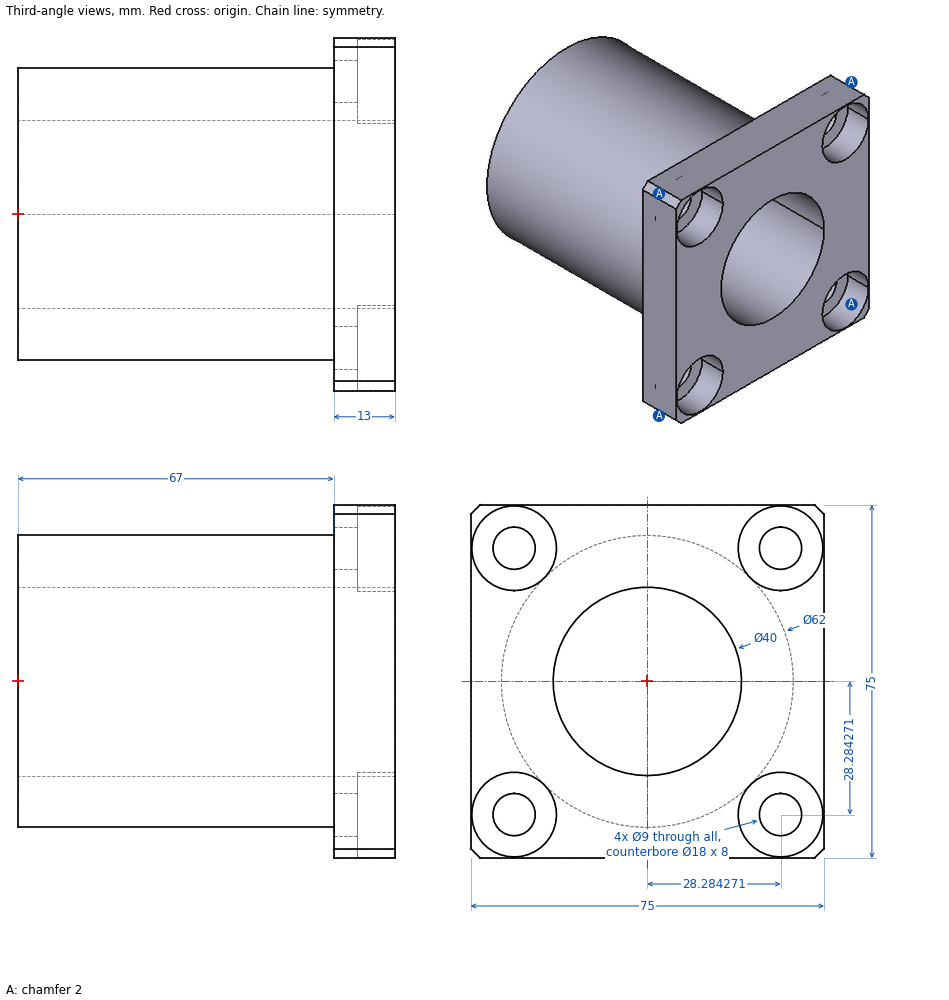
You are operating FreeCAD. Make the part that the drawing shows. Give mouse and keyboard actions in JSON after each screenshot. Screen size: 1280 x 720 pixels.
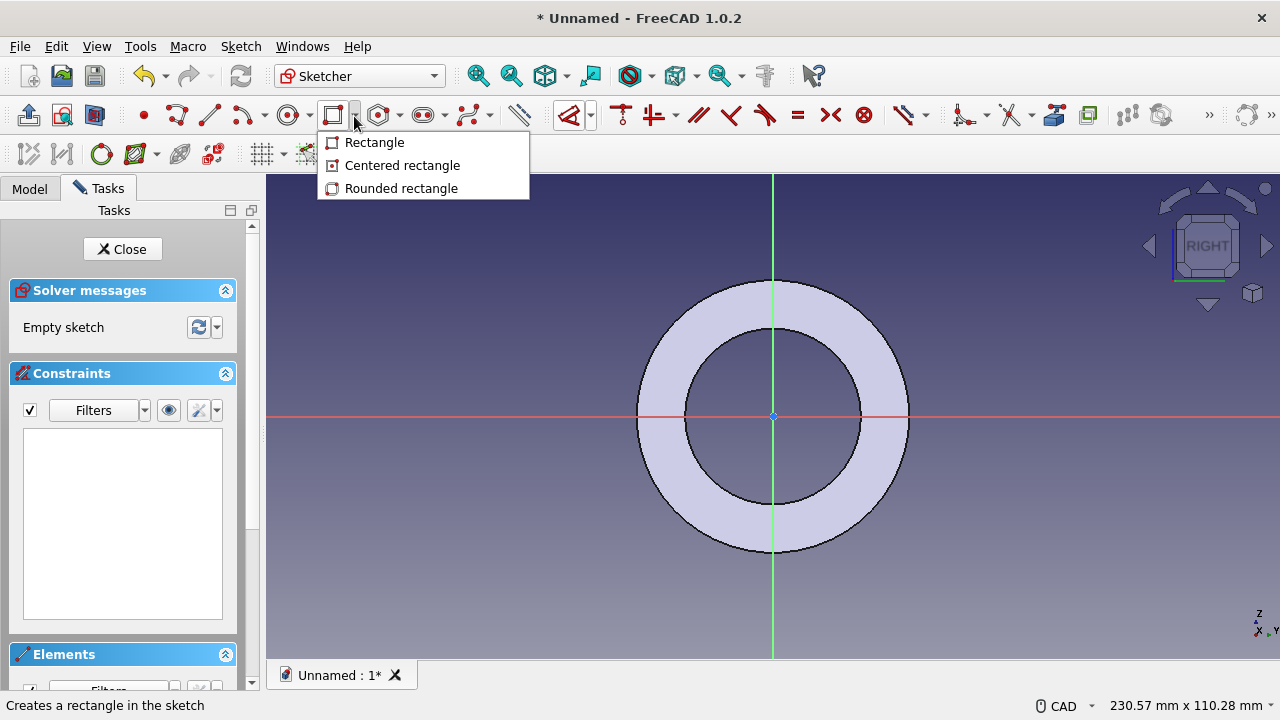
{"action": "left_click", "coordinate": [424, 166]}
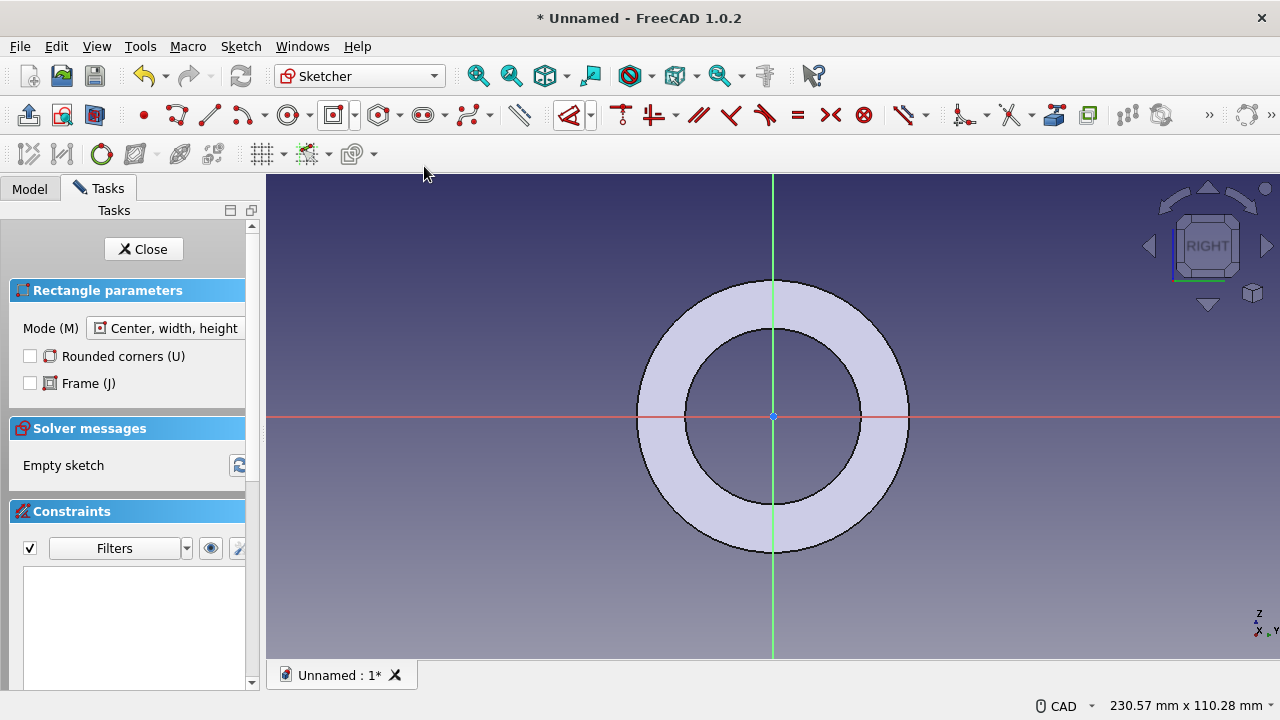
{"action": "left_click", "coordinate": [773, 416]}
{"action": "left_click", "coordinate": [938, 252]}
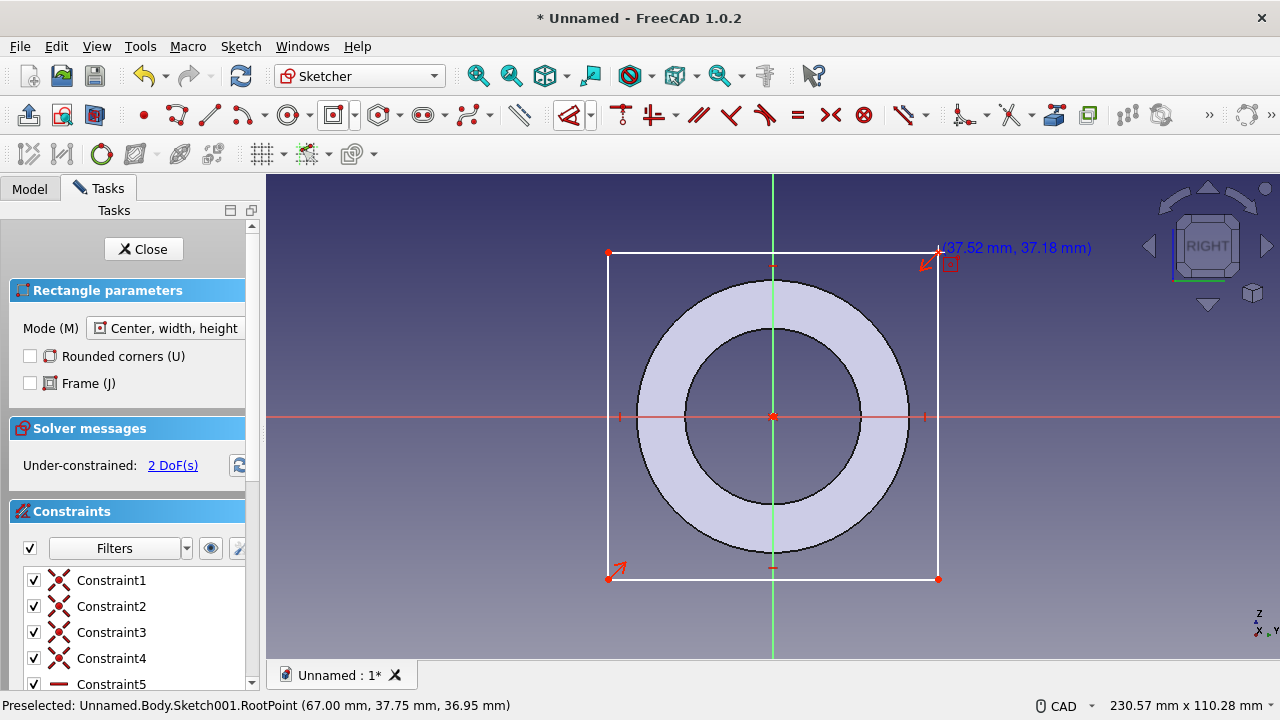
{"action": "left_click", "coordinate": [288, 116]}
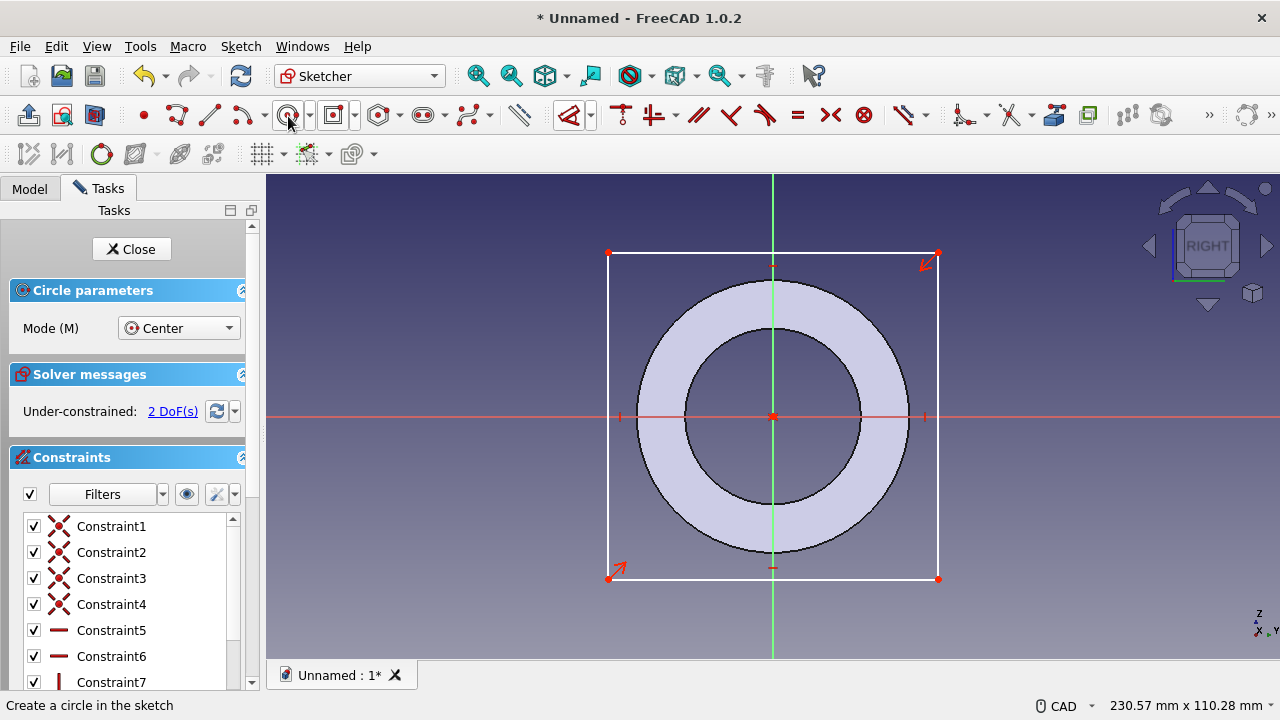
{"action": "left_click", "coordinate": [773, 416]}
{"action": "left_click", "coordinate": [835, 354]}
{"action": "key", "text": "Escape"}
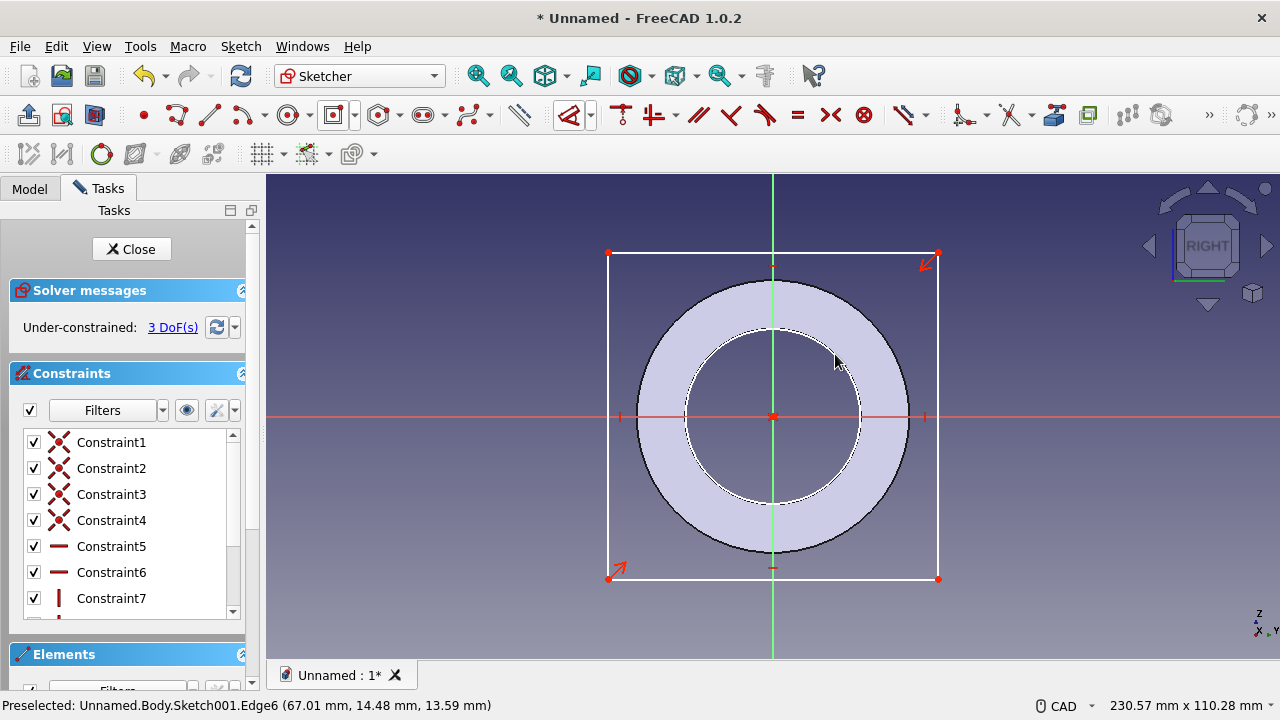
{"action": "left_click", "coordinate": [835, 355]}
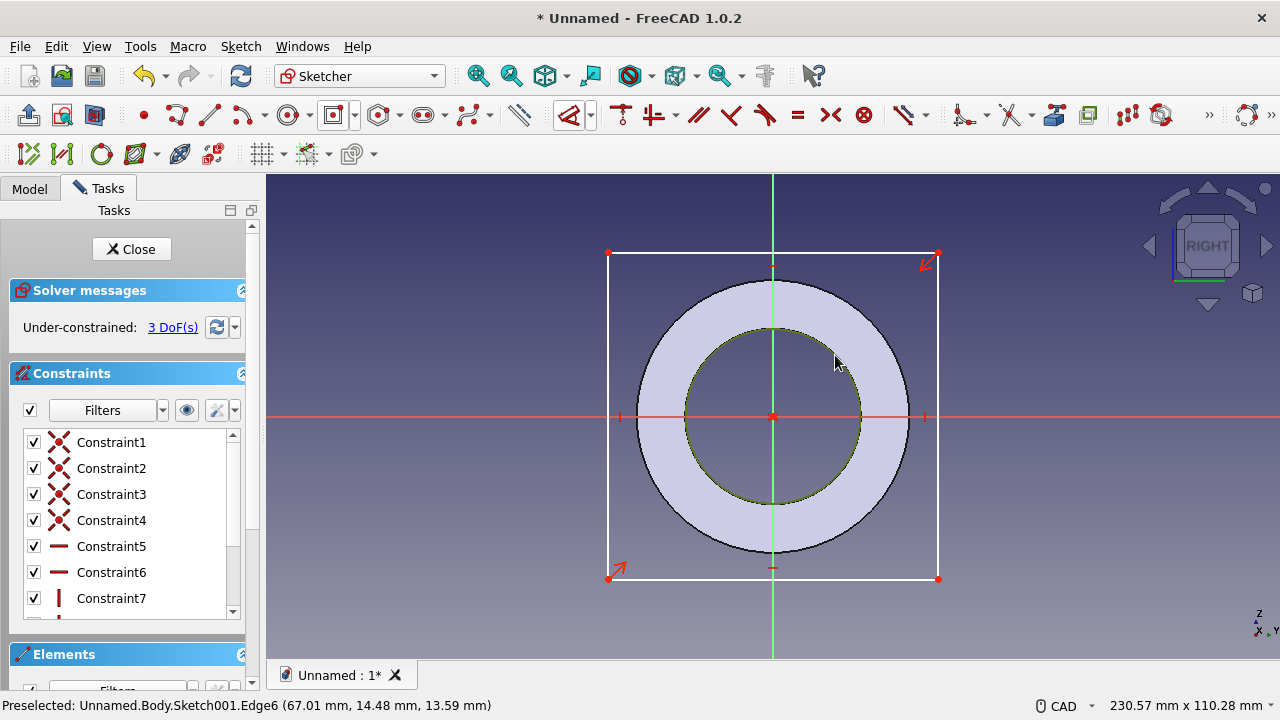
{"action": "left_click", "coordinate": [590, 116]}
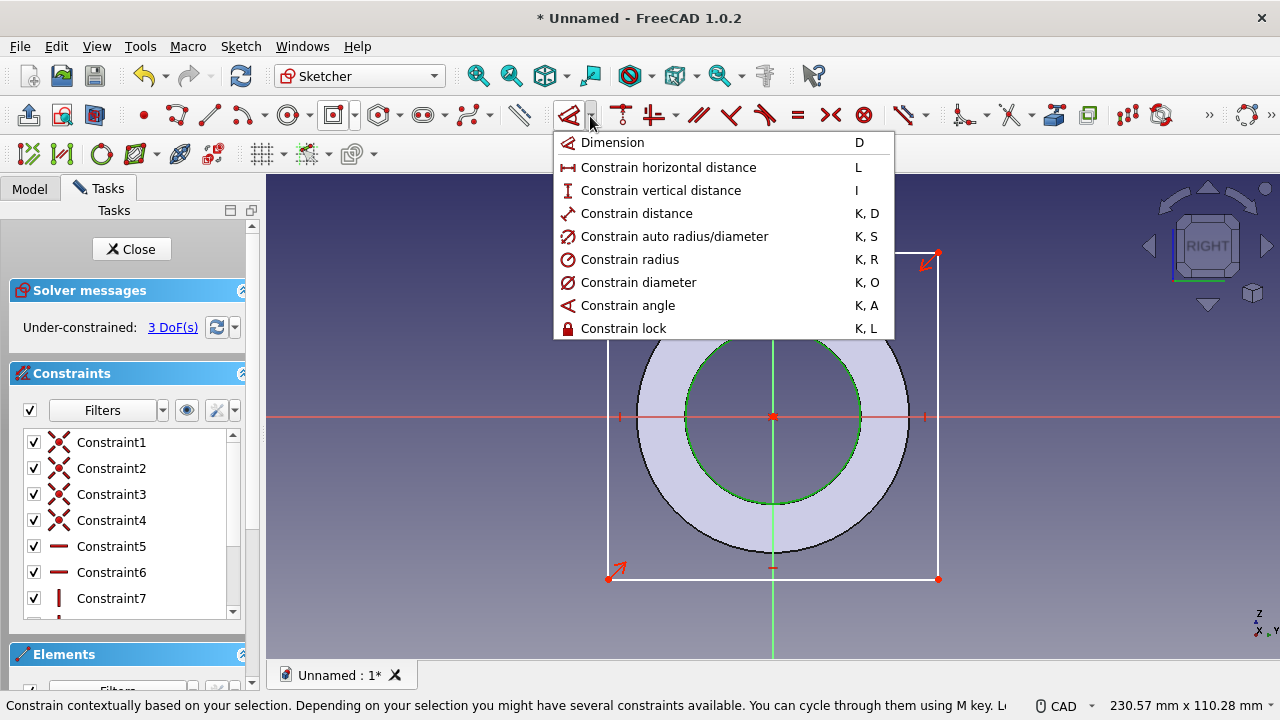
{"action": "left_click", "coordinate": [724, 282]}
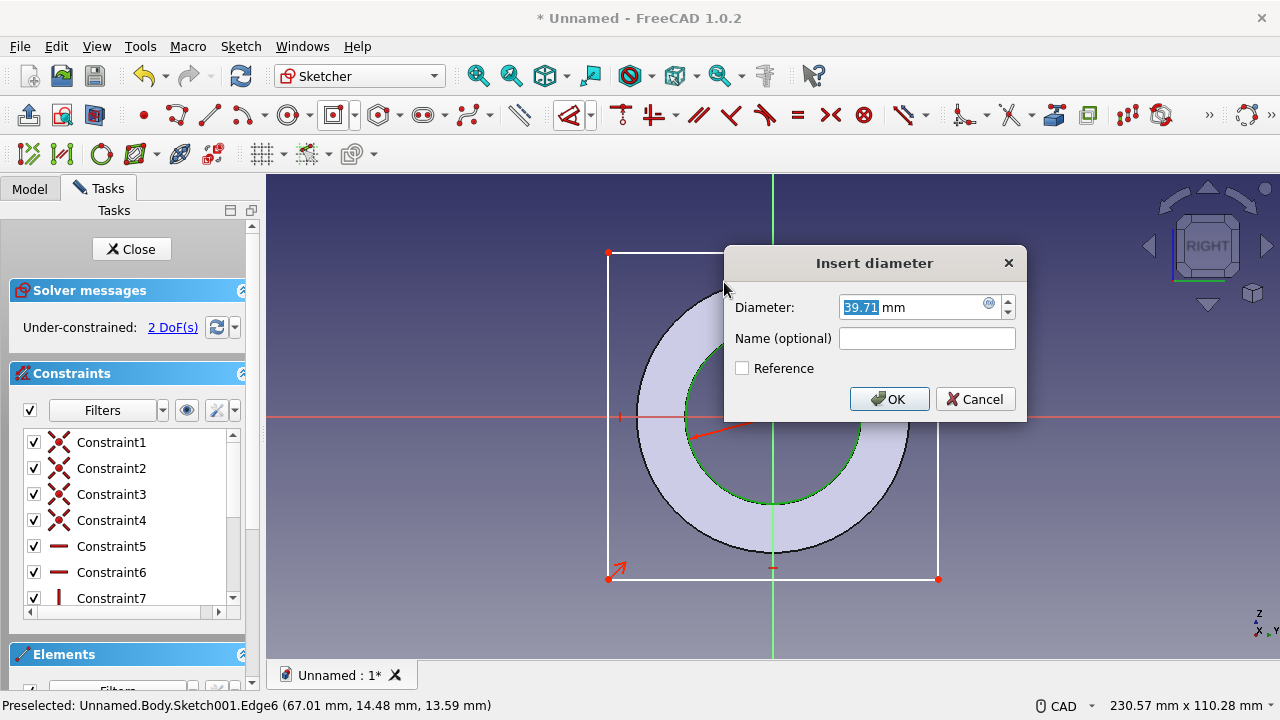
{"action": "type", "text": "40"}
{"action": "key", "text": "Return"}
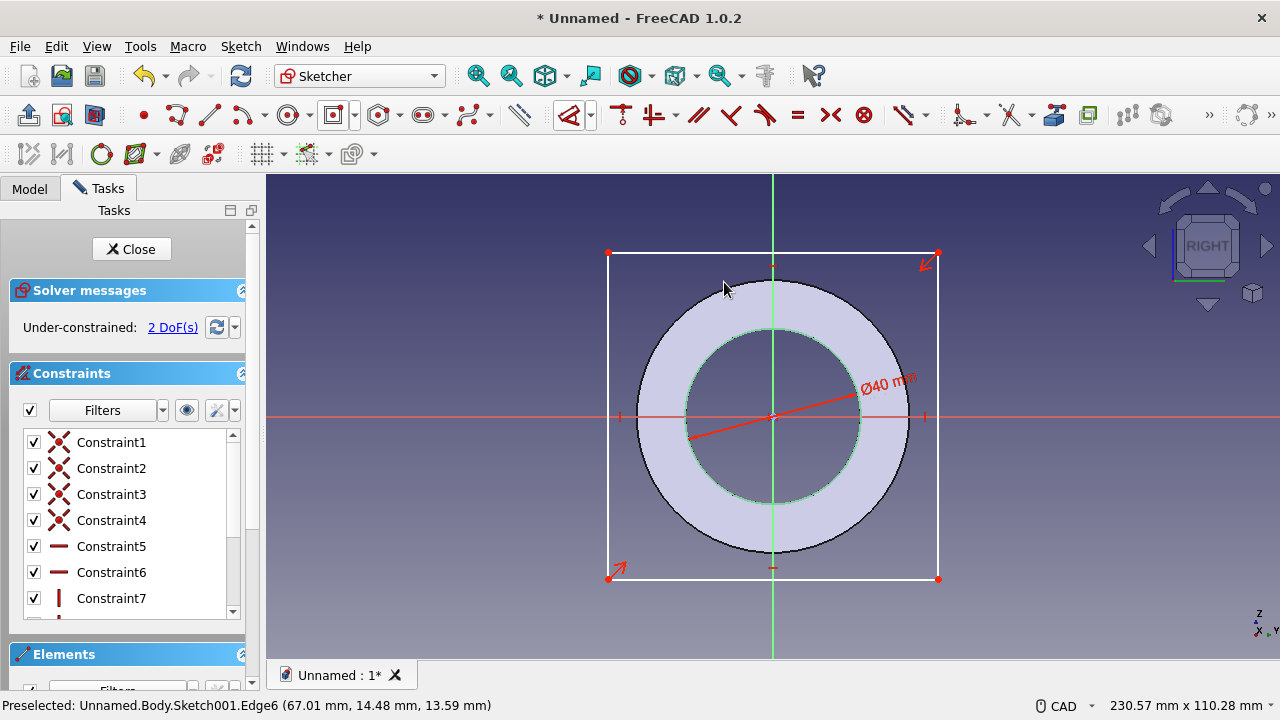
{"action": "left_click", "coordinate": [707, 580]}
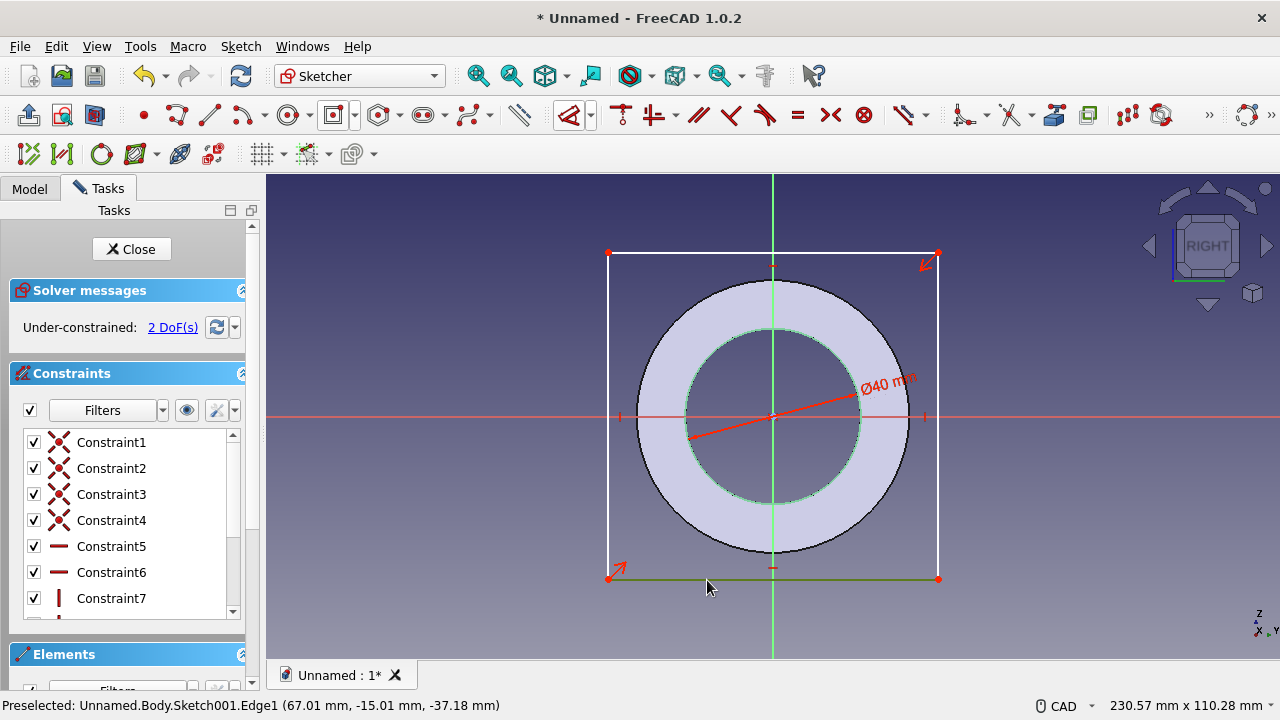
{"action": "key", "text": "l"}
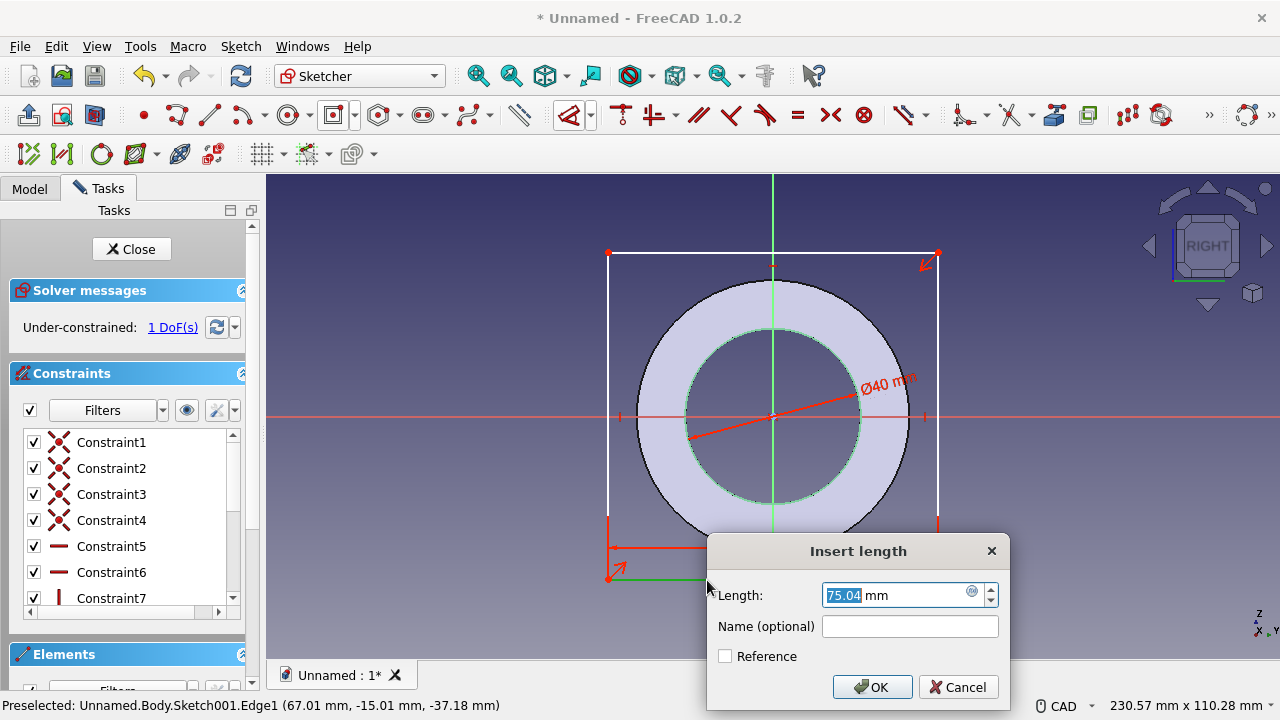
{"action": "type", "text": "75"}
{"action": "key", "text": "Return"}